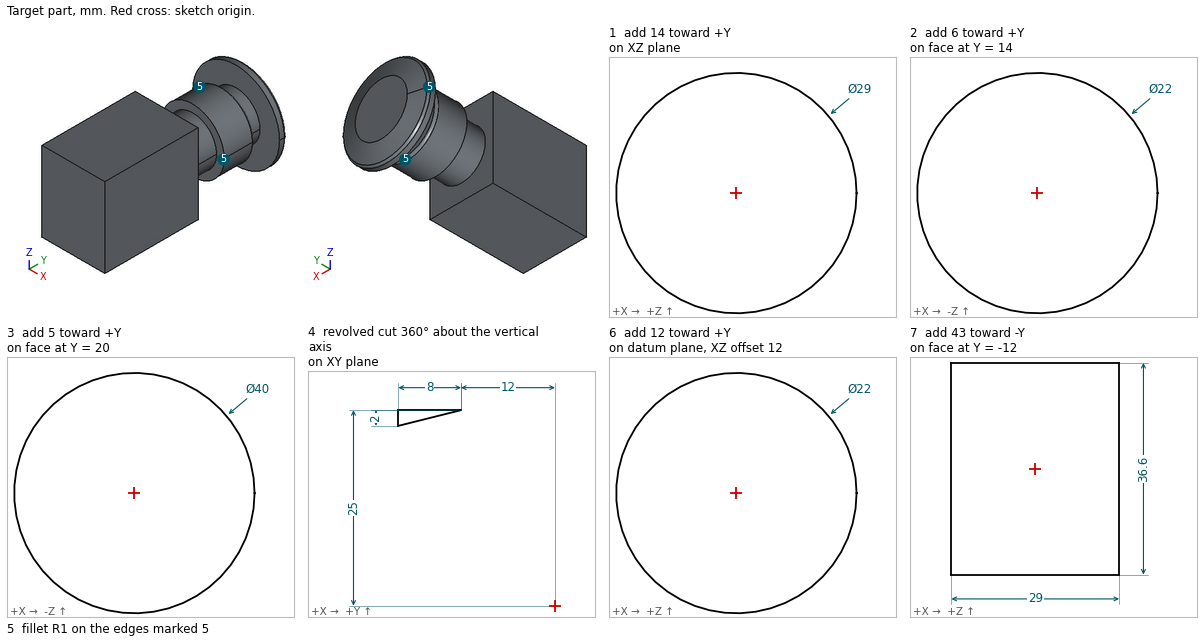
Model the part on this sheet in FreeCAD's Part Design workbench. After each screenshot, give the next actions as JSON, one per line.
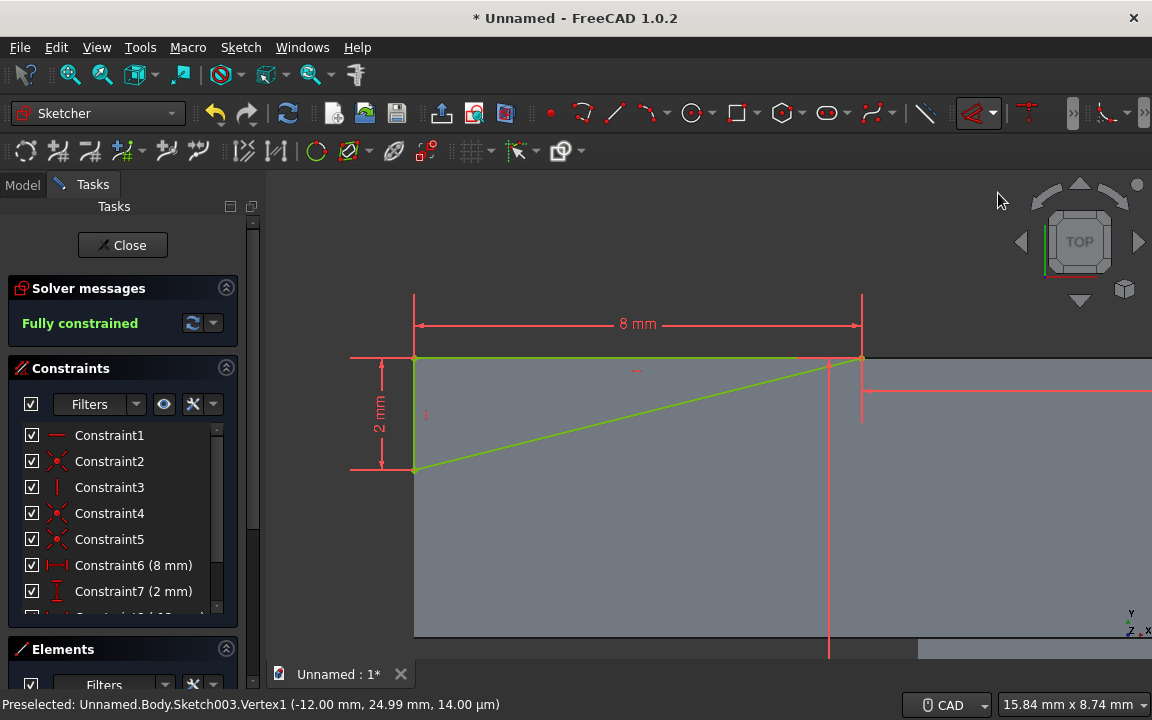
{"action": "left_click", "coordinate": [123, 245]}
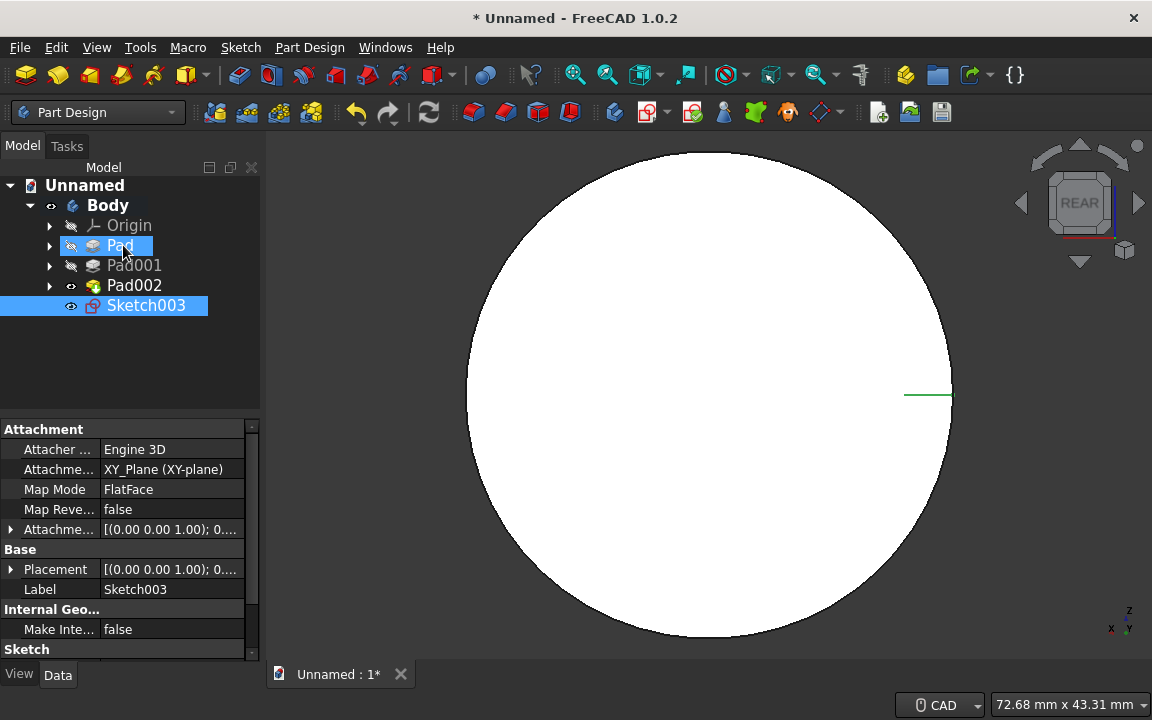
{"action": "left_click", "coordinate": [304, 76]}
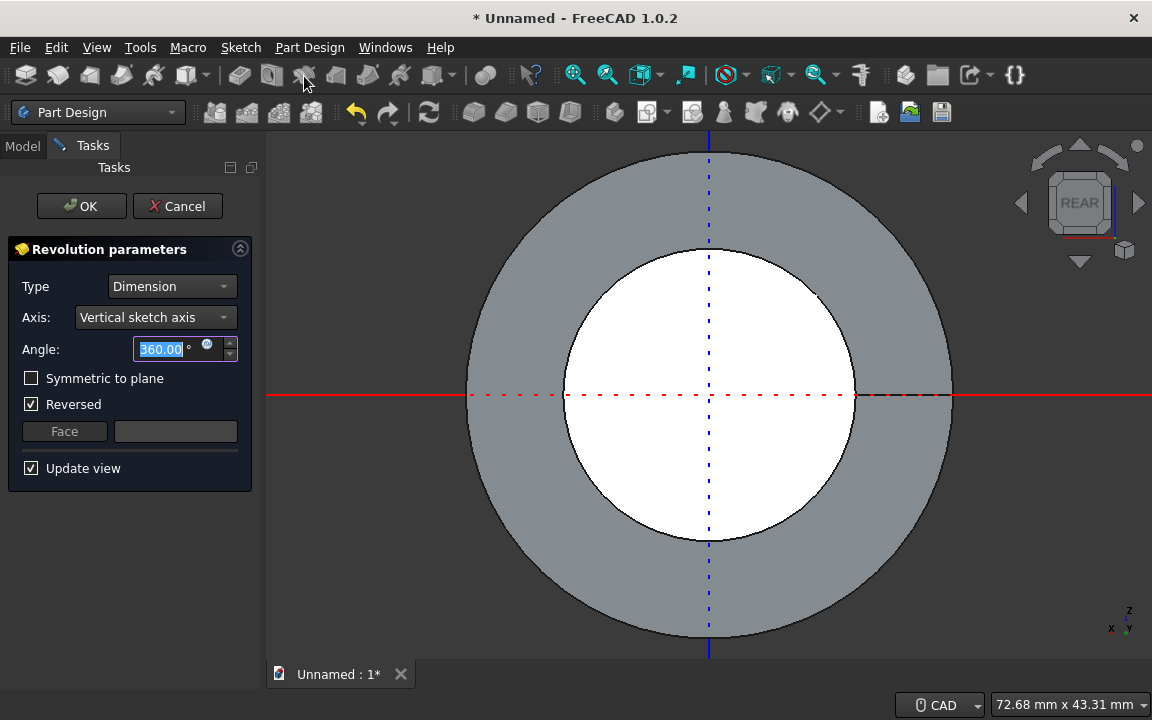
{"action": "left_click", "coordinate": [82, 206]}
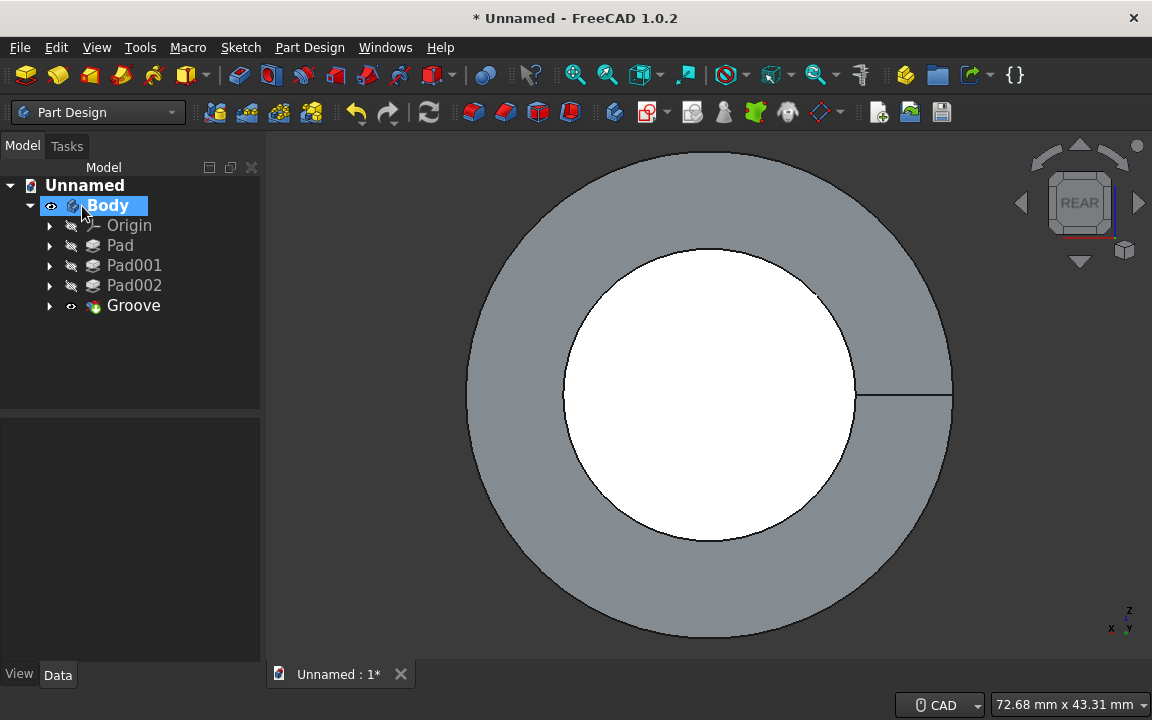
{"action": "key", "text": "0"}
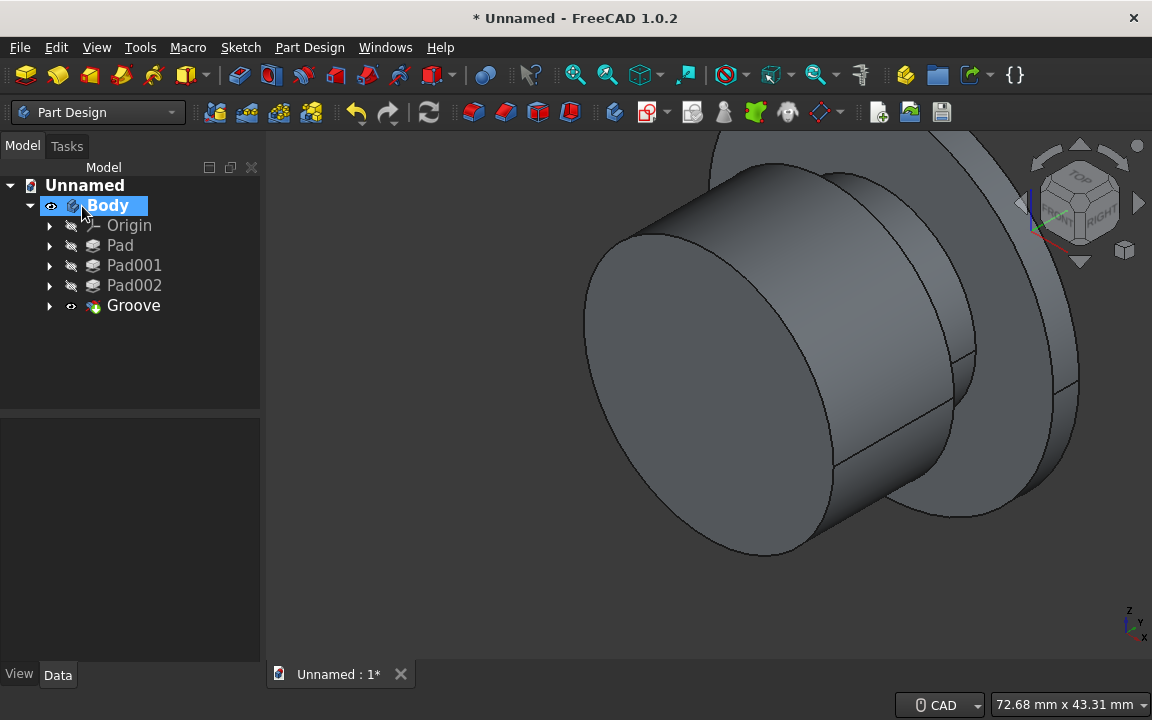
{"action": "key", "text": "v f"}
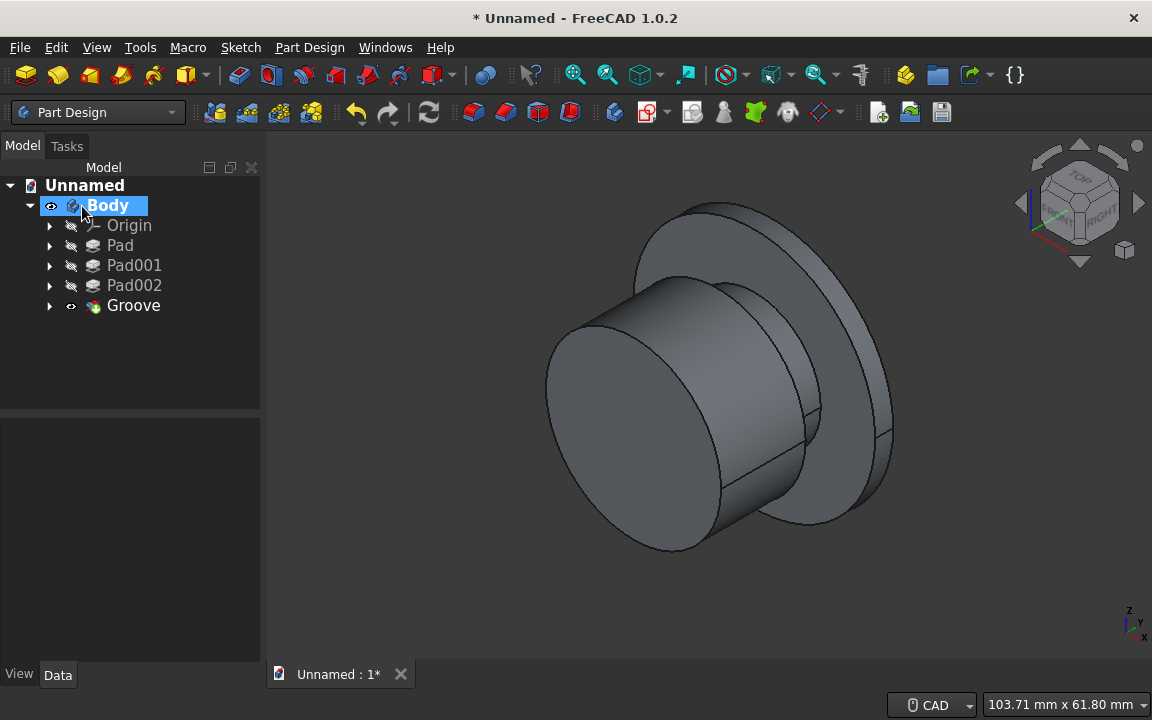
{"action": "key", "text": "2"}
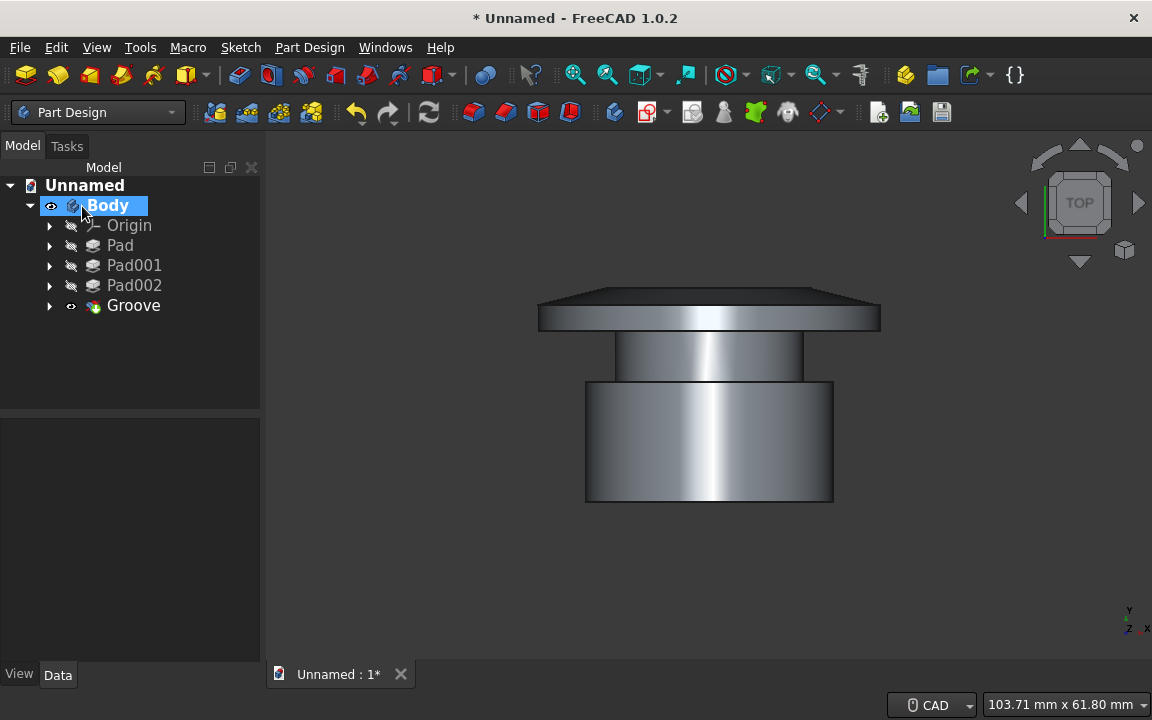
{"action": "left_click", "coordinate": [576, 76]}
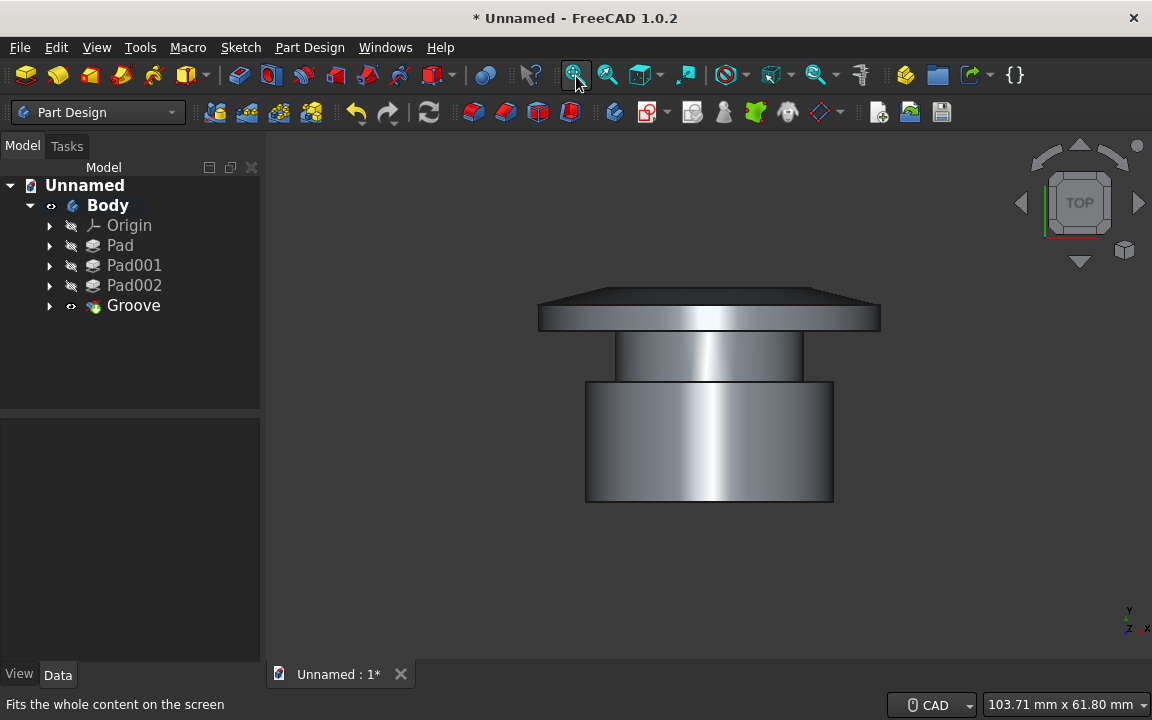
{"action": "left_click", "coordinate": [709, 304]}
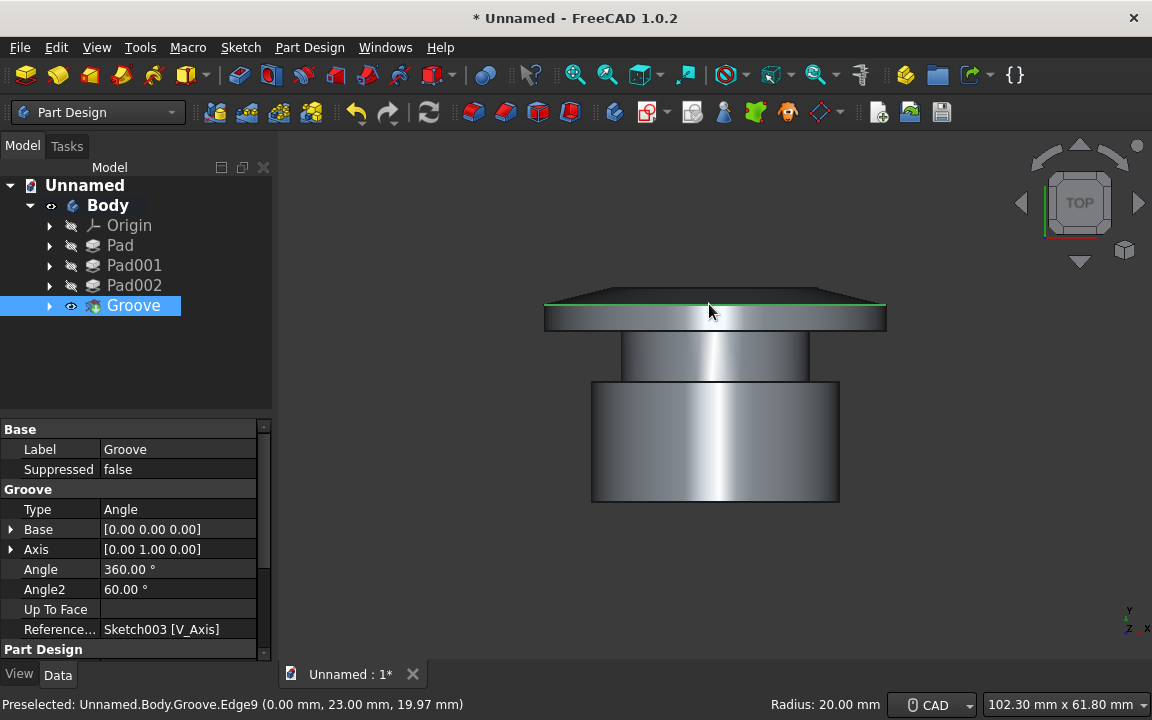
{"action": "left_click", "coordinate": [615, 381], "text": "ctrl"}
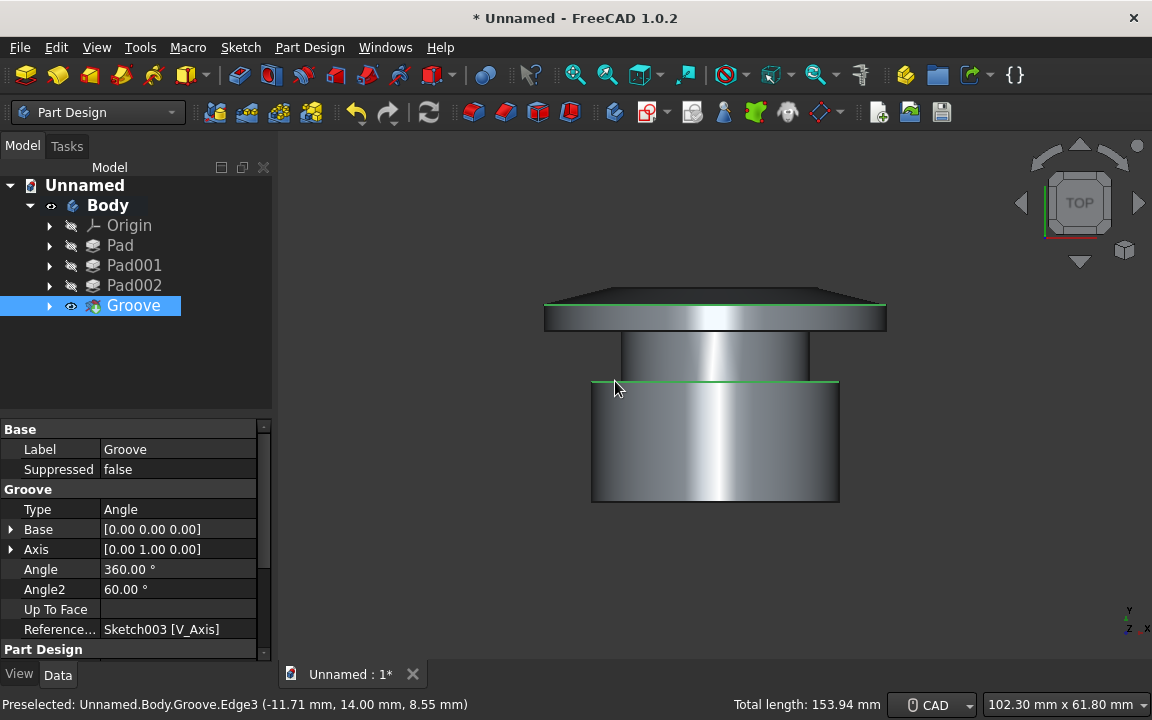
{"action": "left_click", "coordinate": [474, 112]}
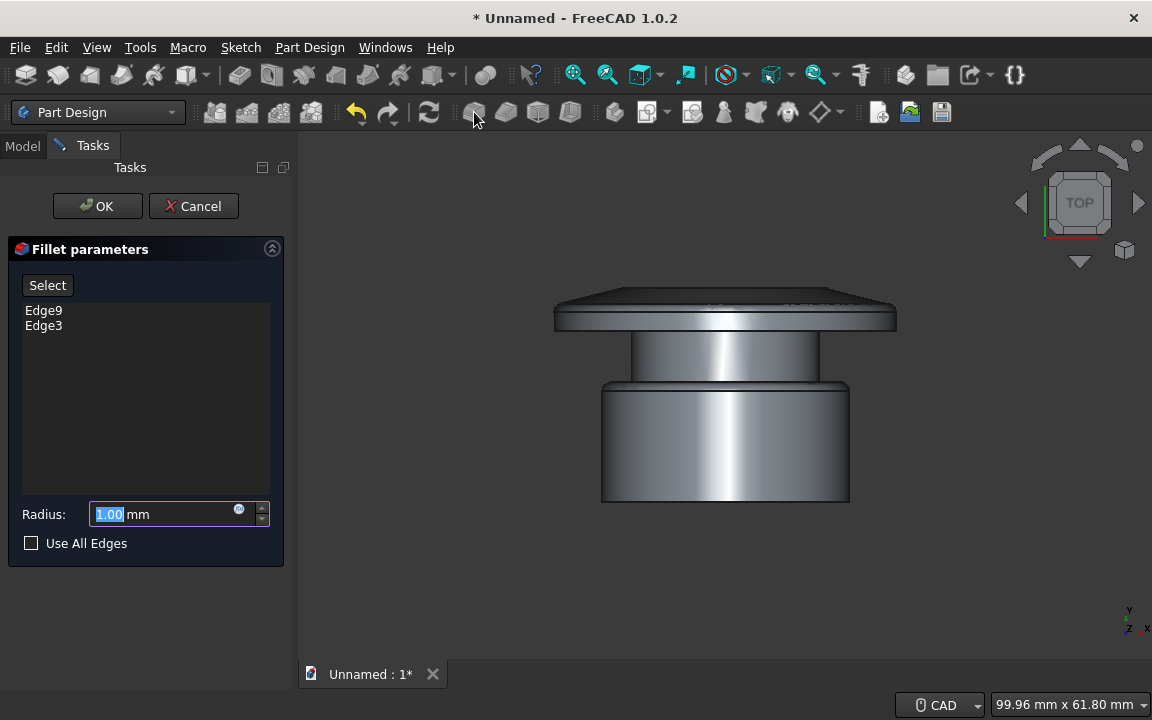
{"action": "type", "text": "1"}
{"action": "key", "text": "Tab"}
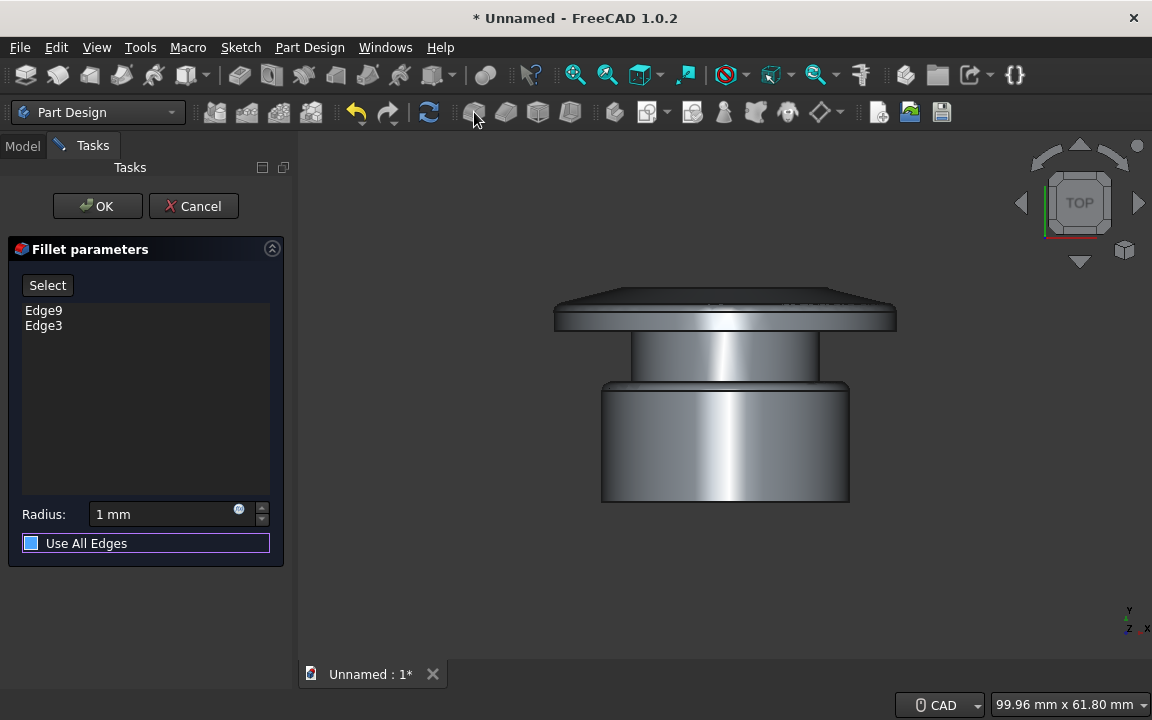
{"action": "left_click", "coordinate": [98, 206]}